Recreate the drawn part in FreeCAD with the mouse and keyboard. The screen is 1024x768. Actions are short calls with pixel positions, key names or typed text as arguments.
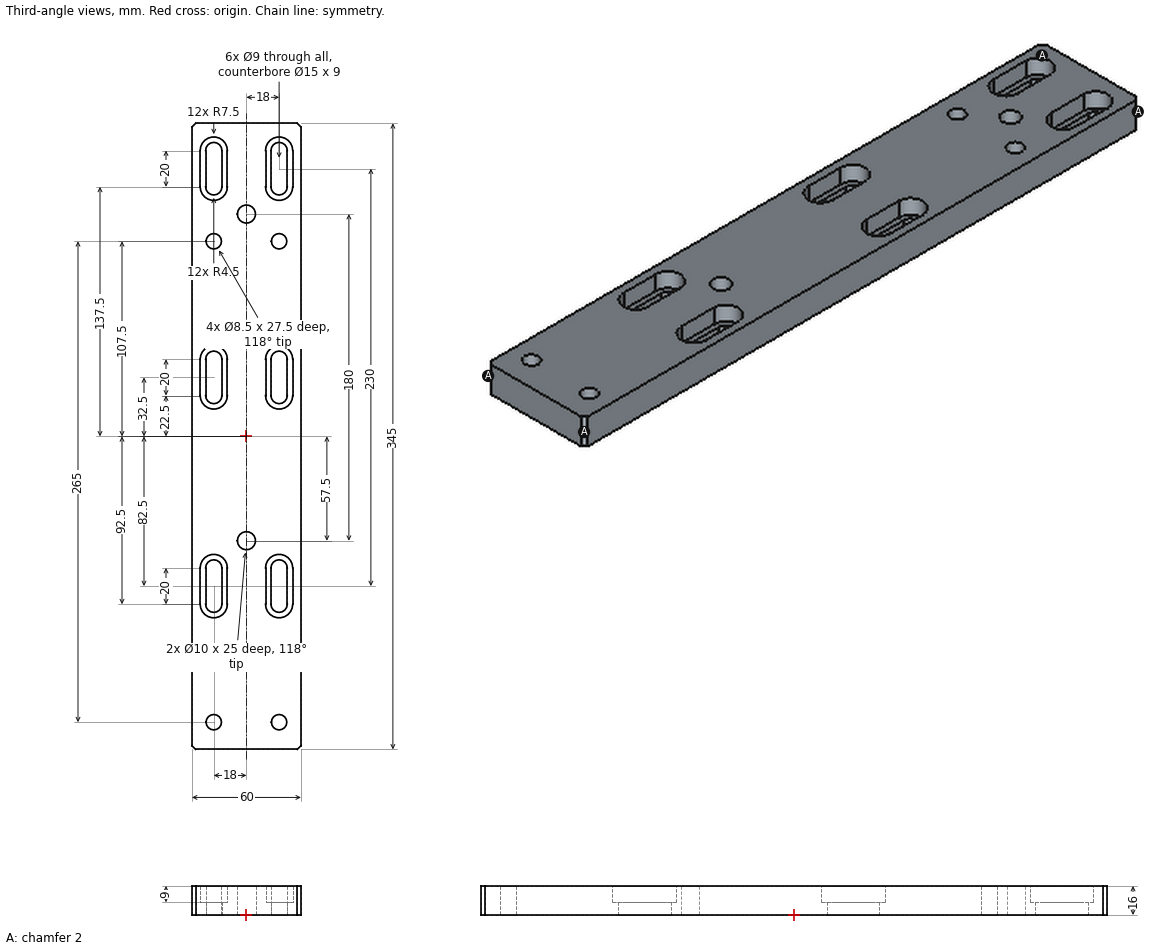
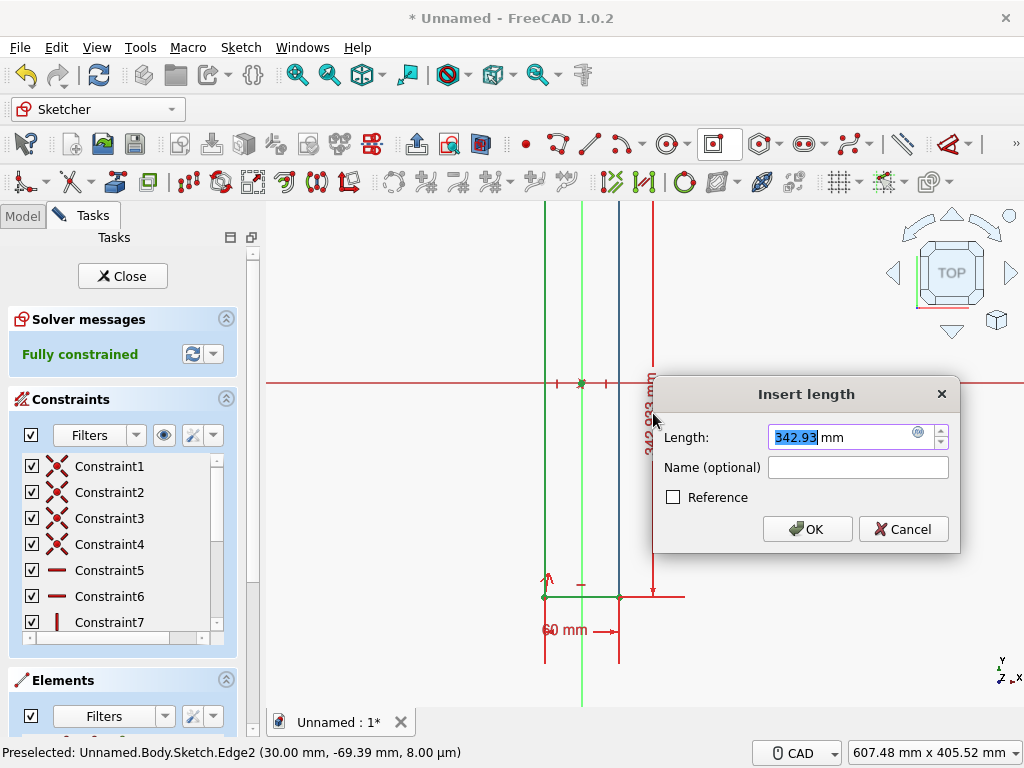
text(345)
key(Return)
key(Escape)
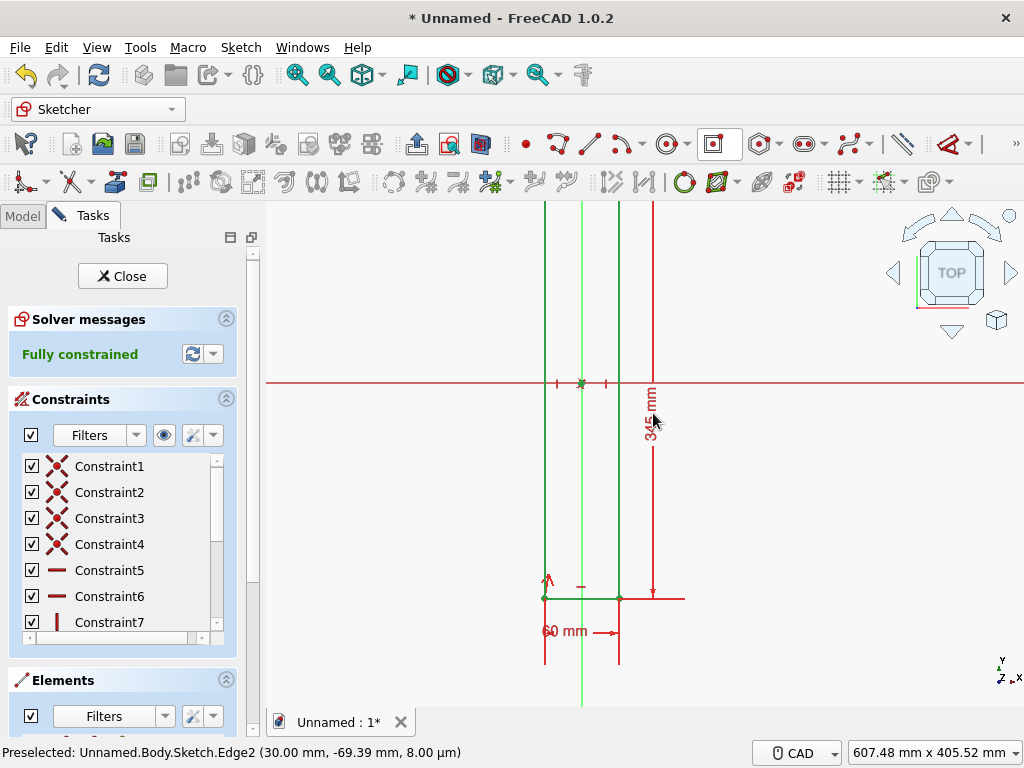
click(123, 276)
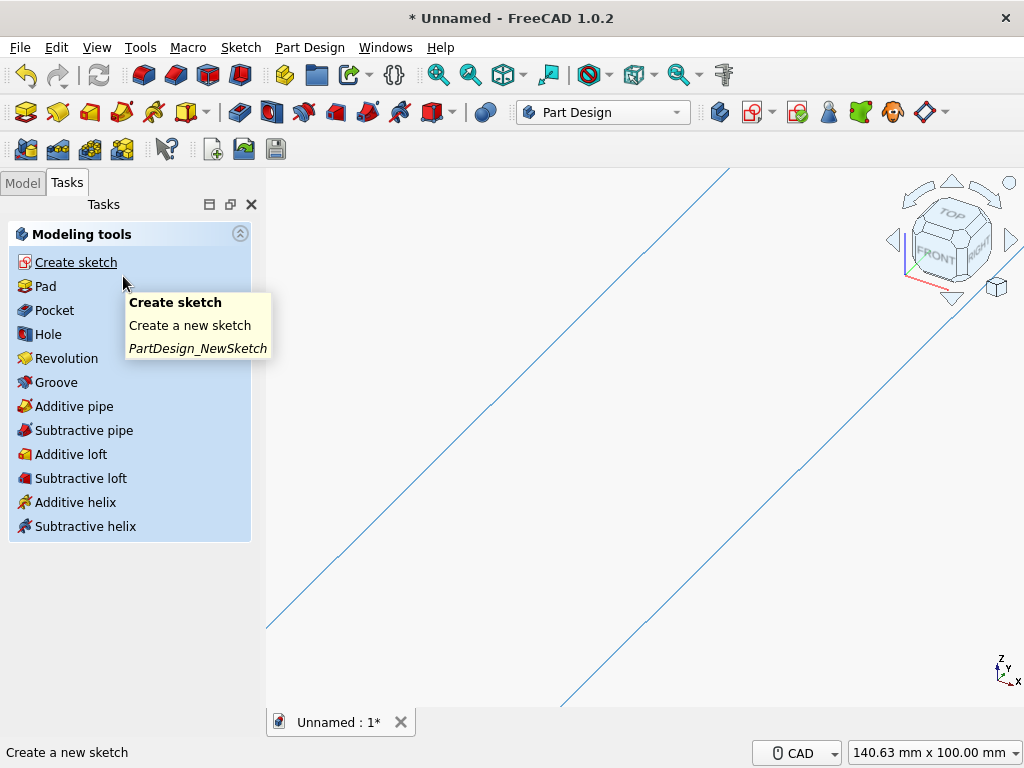
click(26, 112)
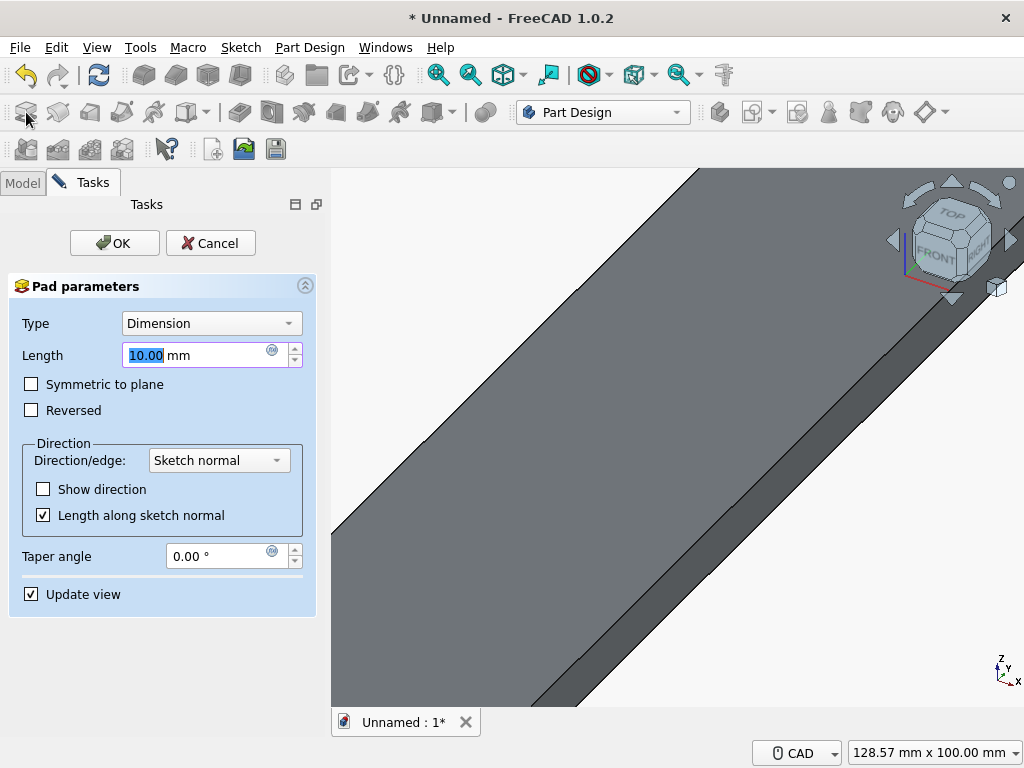
text(16)
key(Tab)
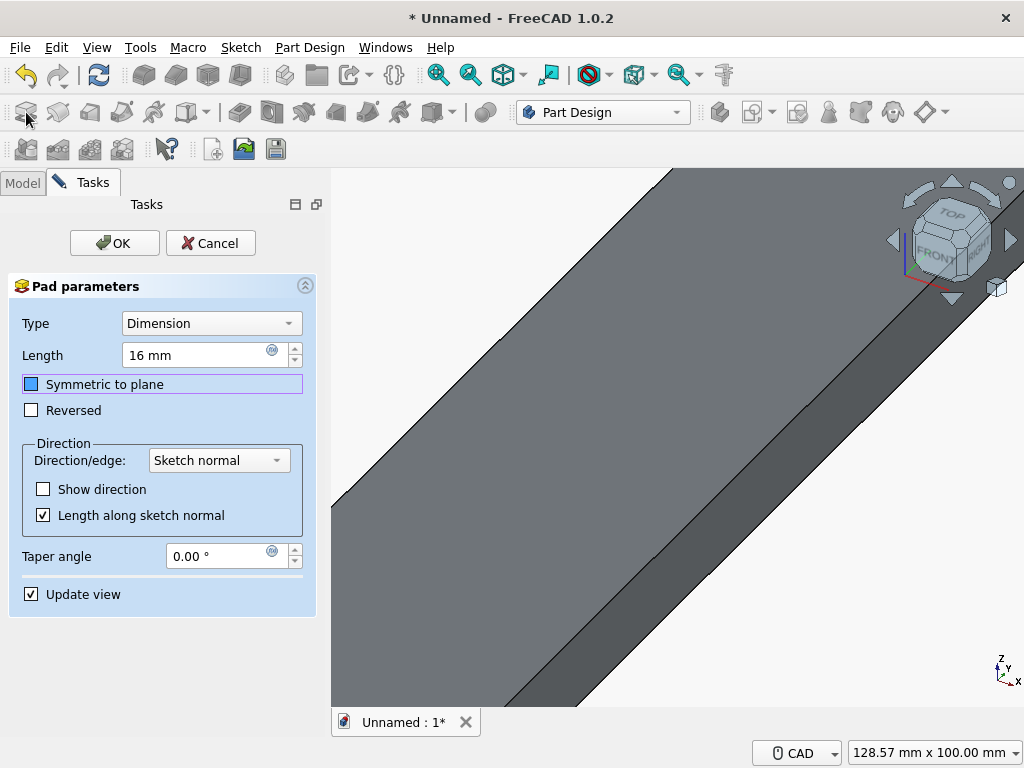
click(115, 243)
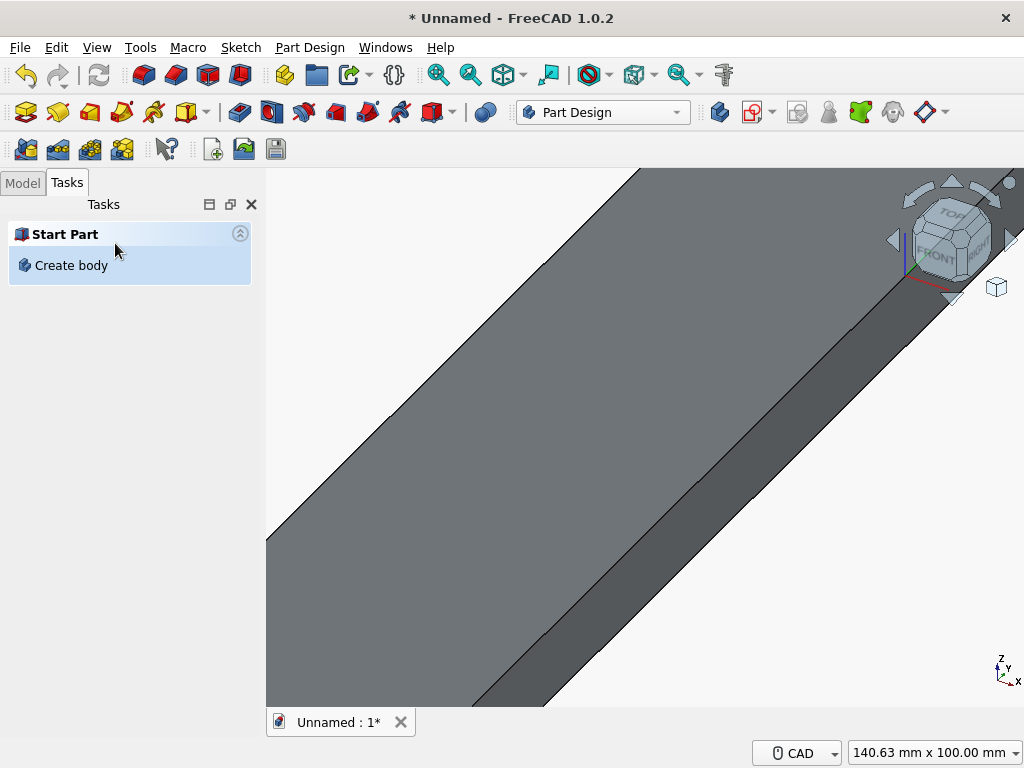
click(440, 76)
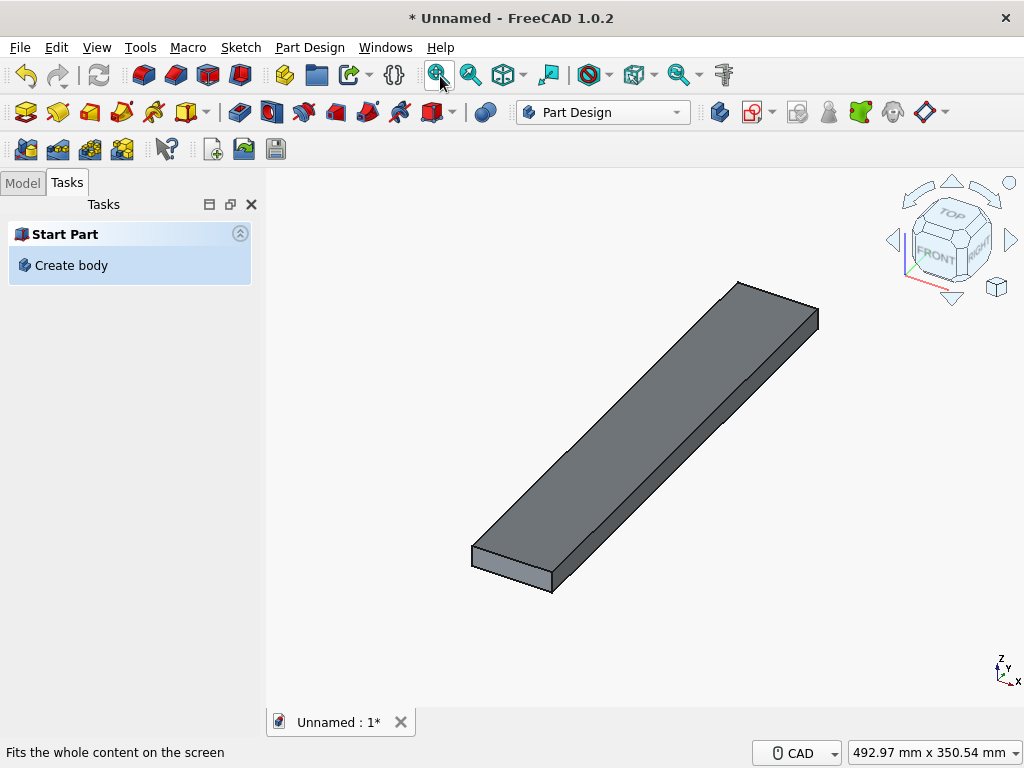
click(721, 351)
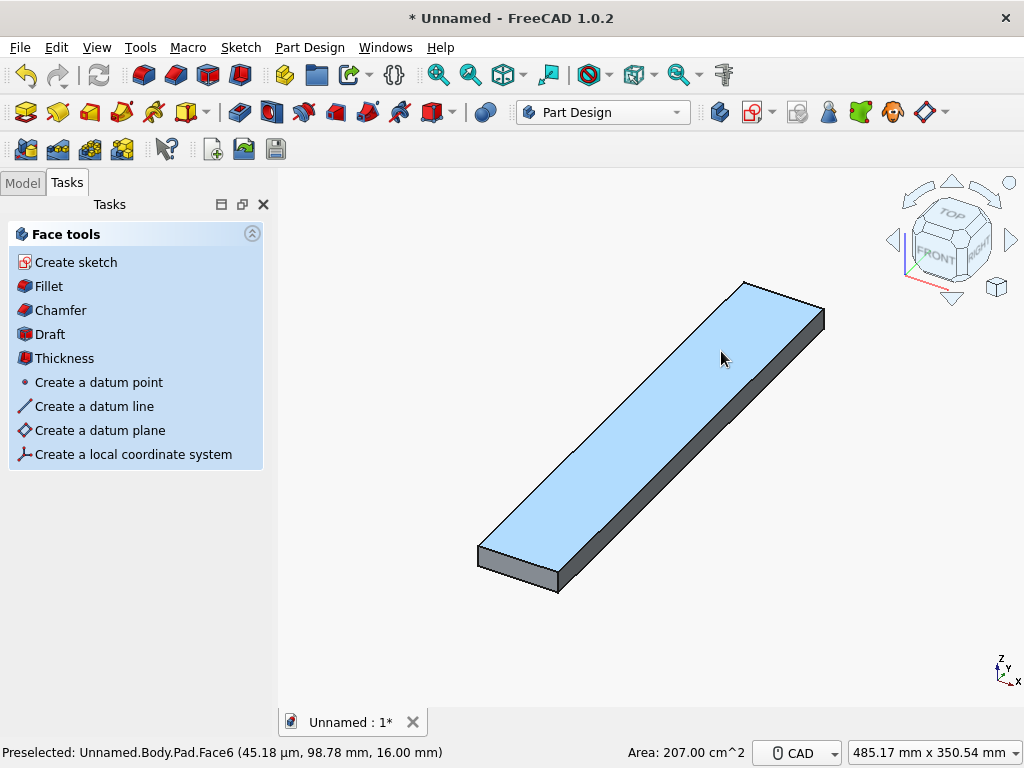
click(752, 112)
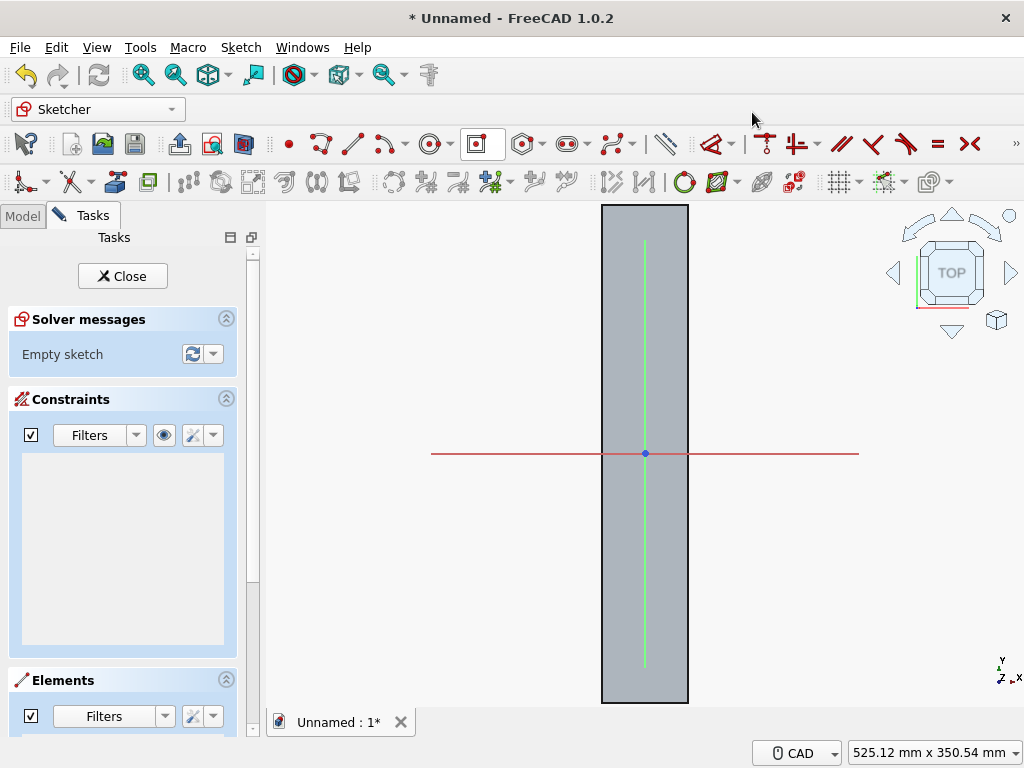
scroll(294, 666, down, 1)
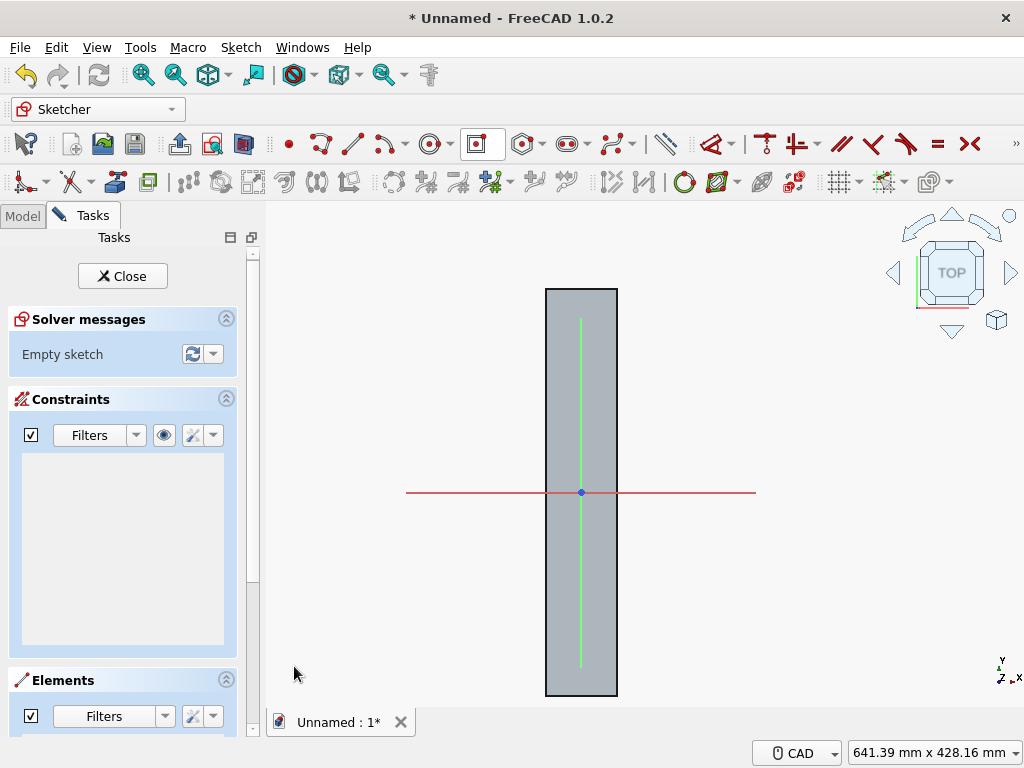
click(430, 144)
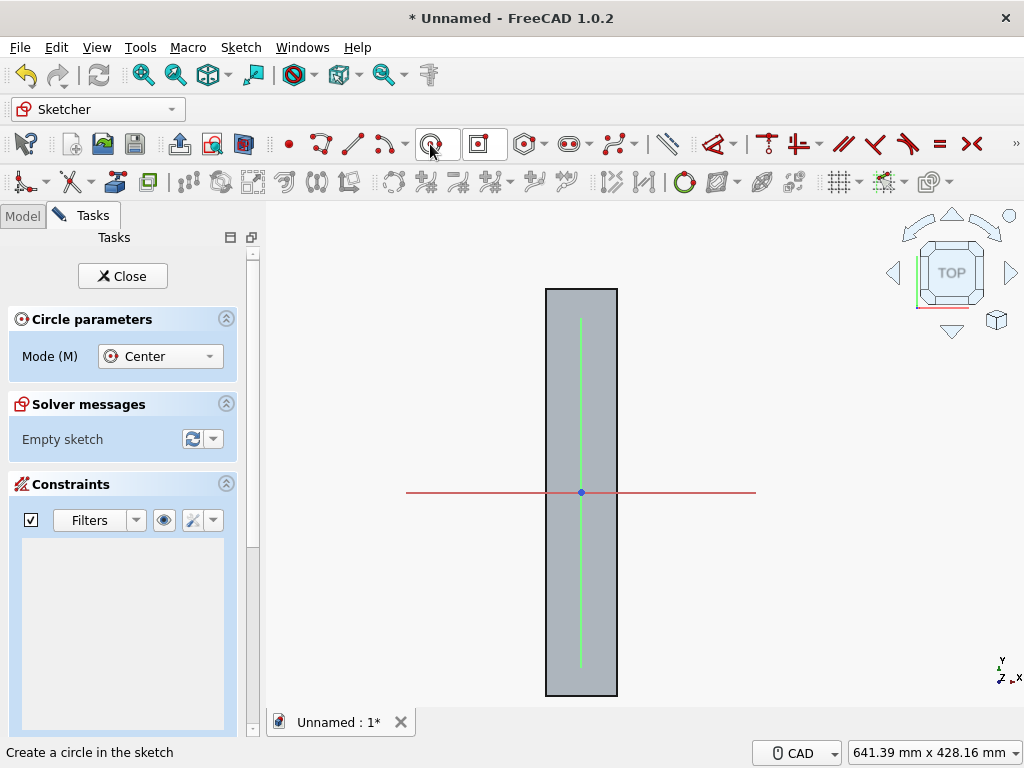
scroll(603, 318, up, 8)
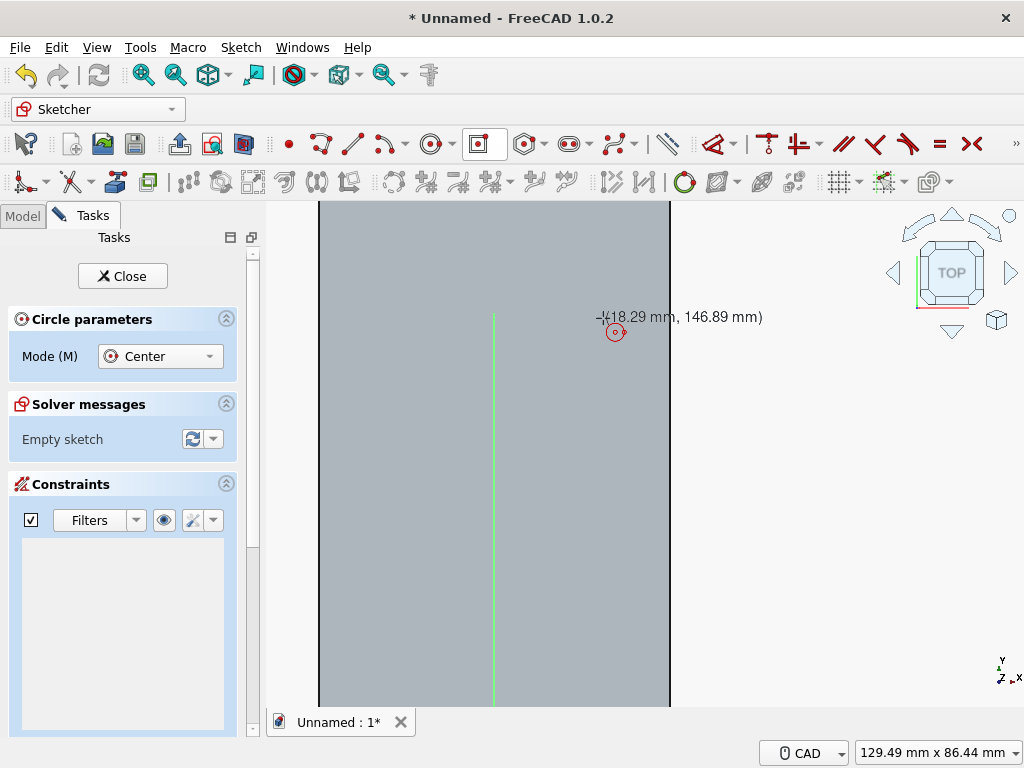
scroll(603, 278, down, 7)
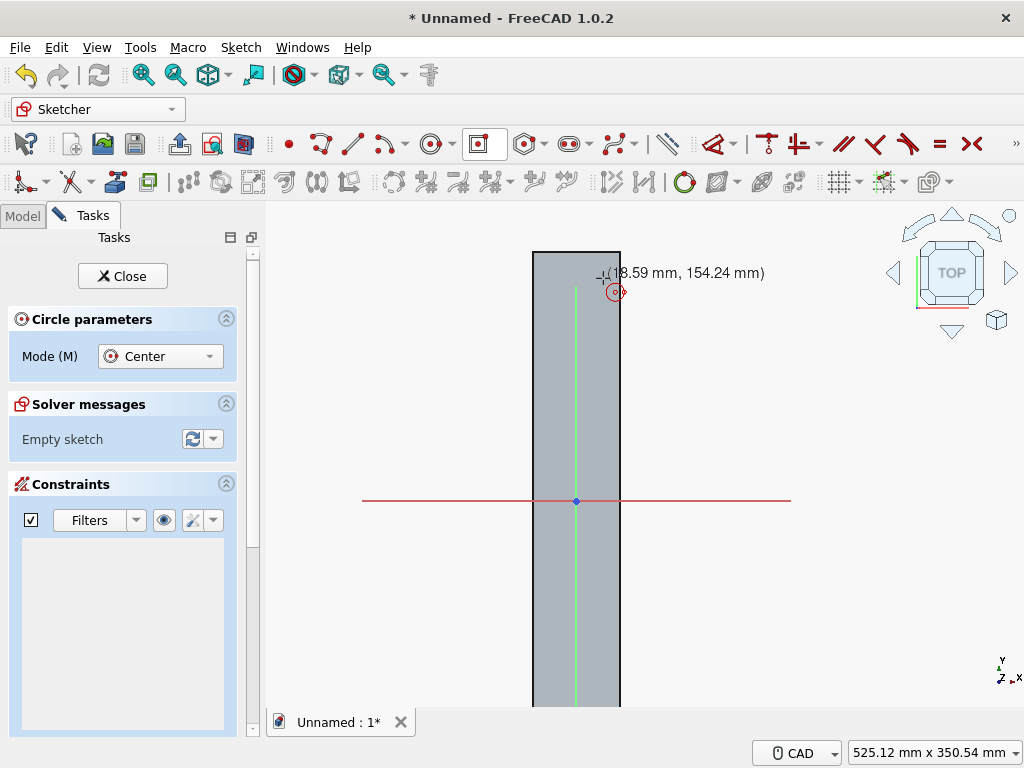
click(602, 288)